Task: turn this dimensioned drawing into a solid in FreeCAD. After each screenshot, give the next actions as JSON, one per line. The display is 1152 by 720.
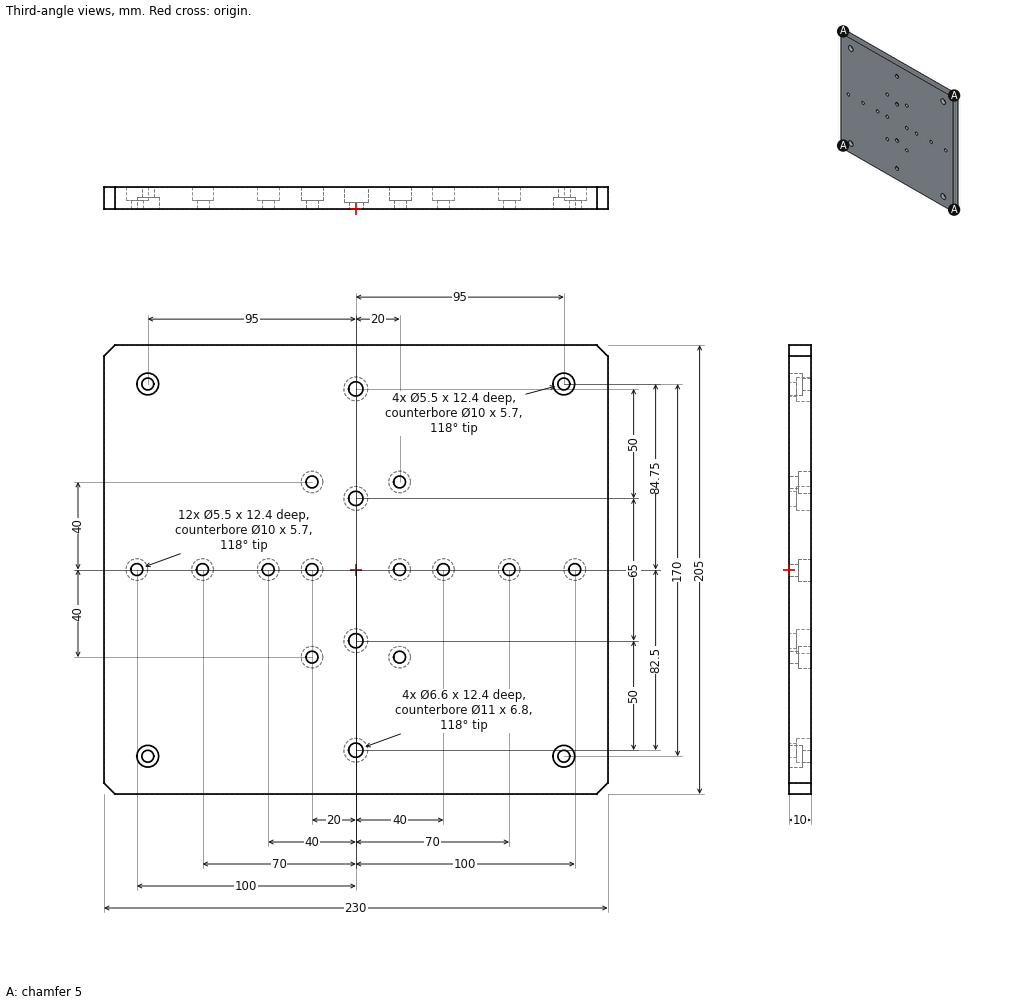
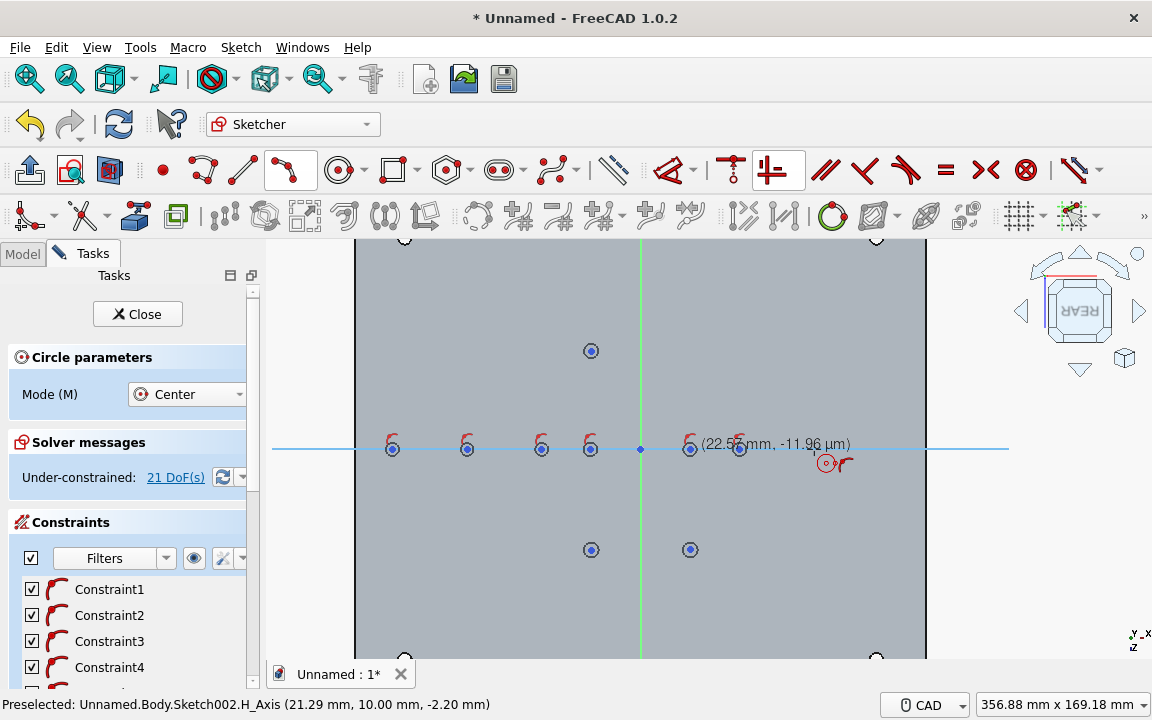
{"action": "left_click", "coordinate": [814, 449]}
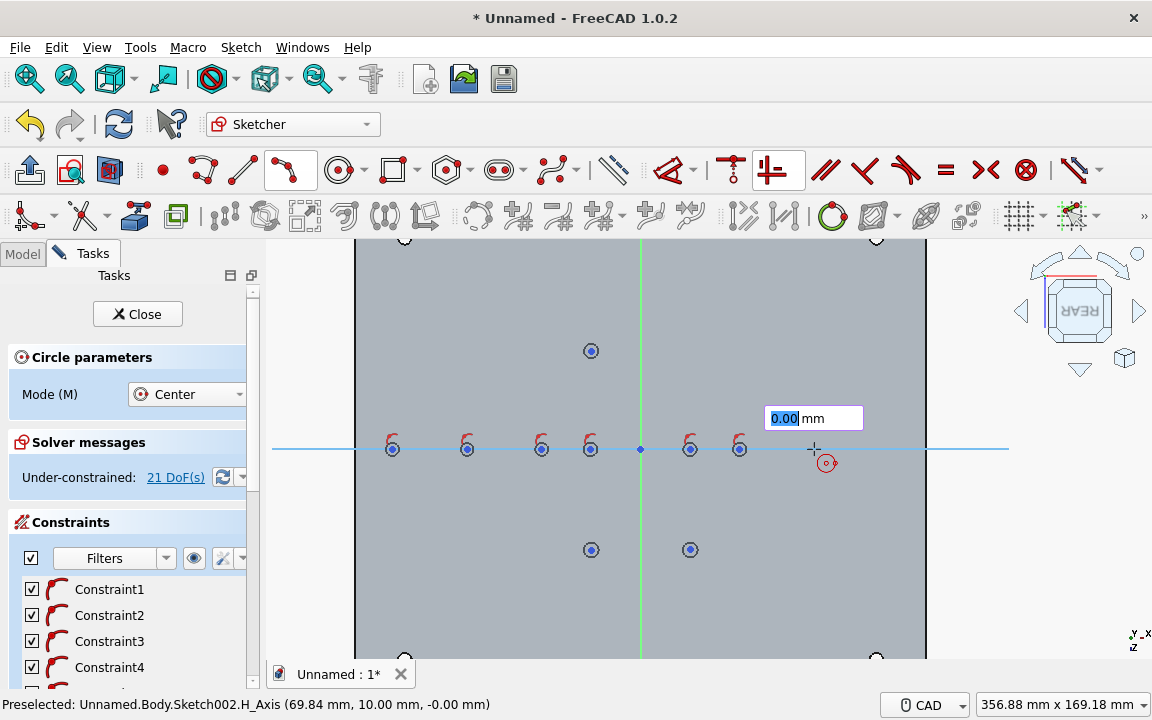
{"action": "scroll", "coordinate": [817, 443], "scroll_direction": "up", "scroll_amount": 5}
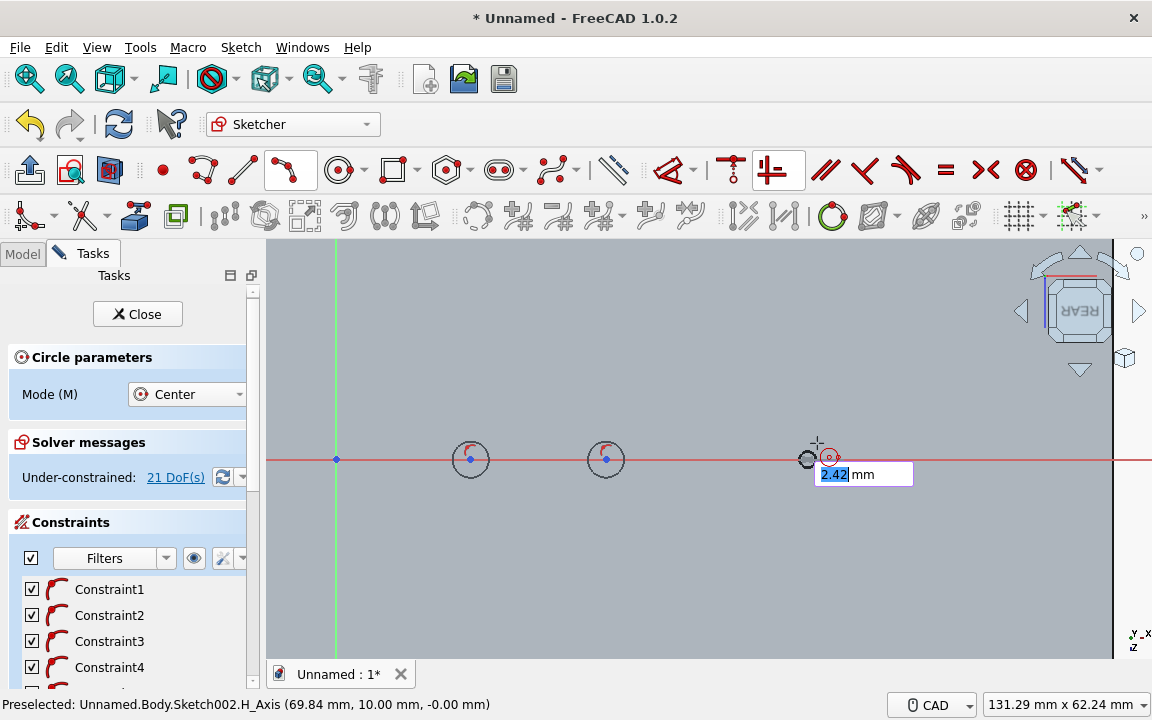
{"action": "left_click", "coordinate": [815, 442]}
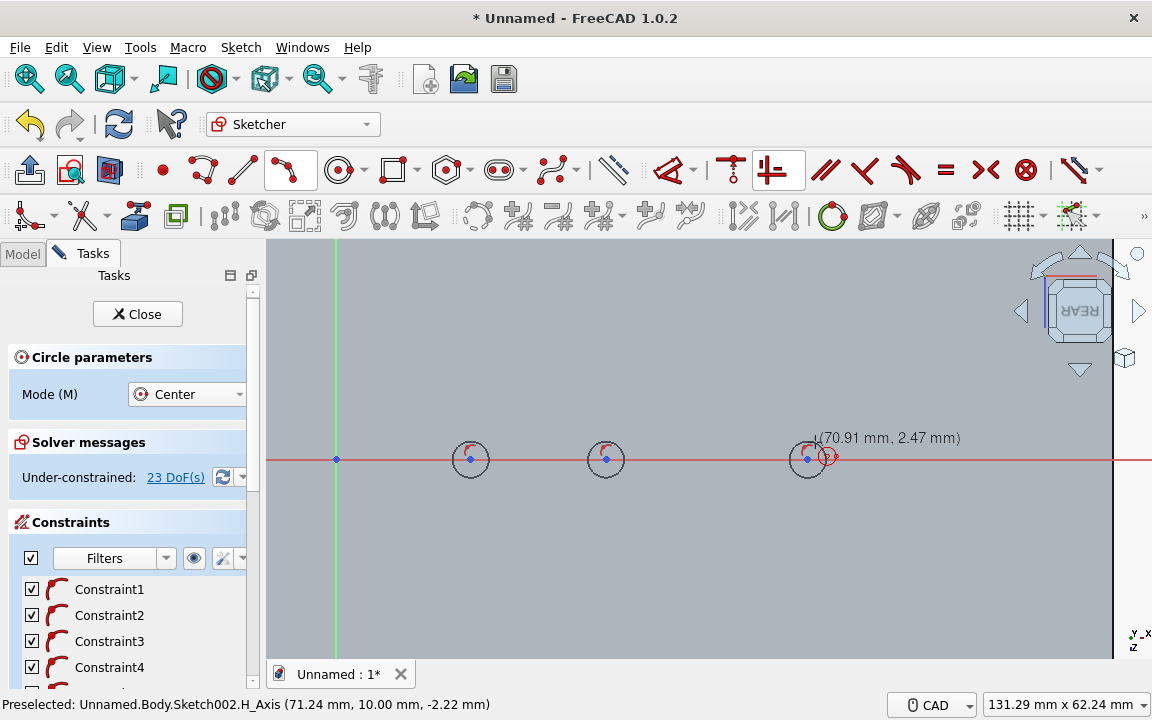
{"action": "scroll", "coordinate": [817, 443], "scroll_direction": "down", "scroll_amount": 5}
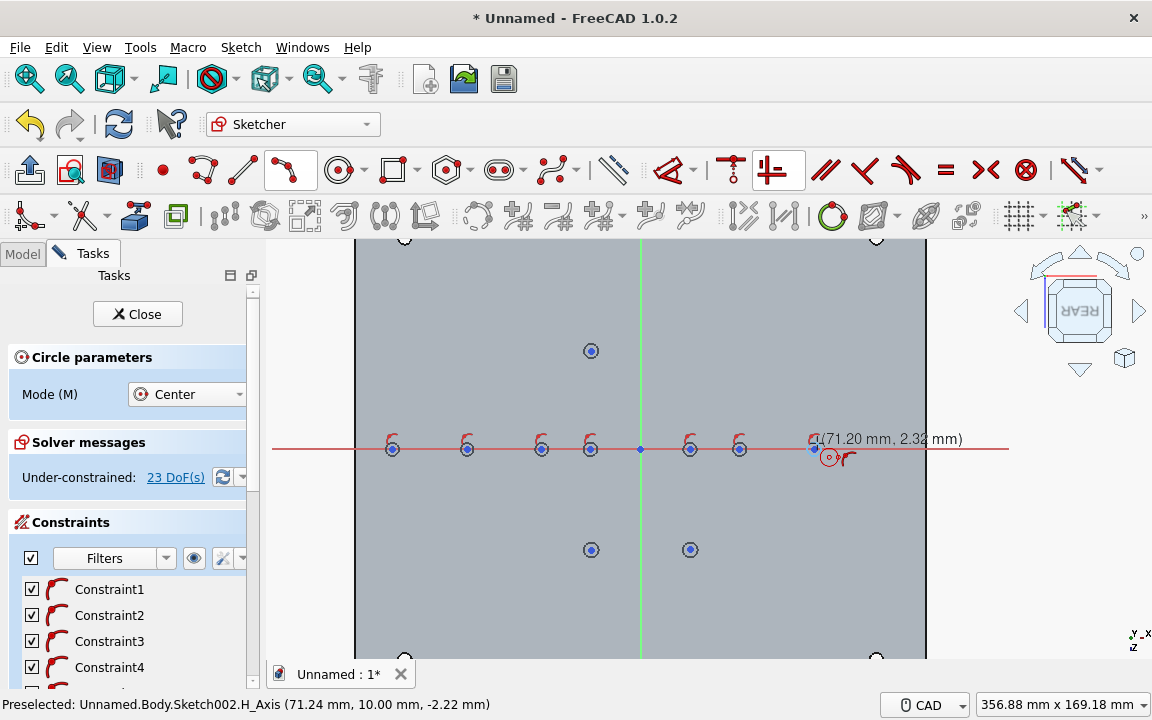
{"action": "scroll", "coordinate": [889, 449], "scroll_direction": "up", "scroll_amount": 7}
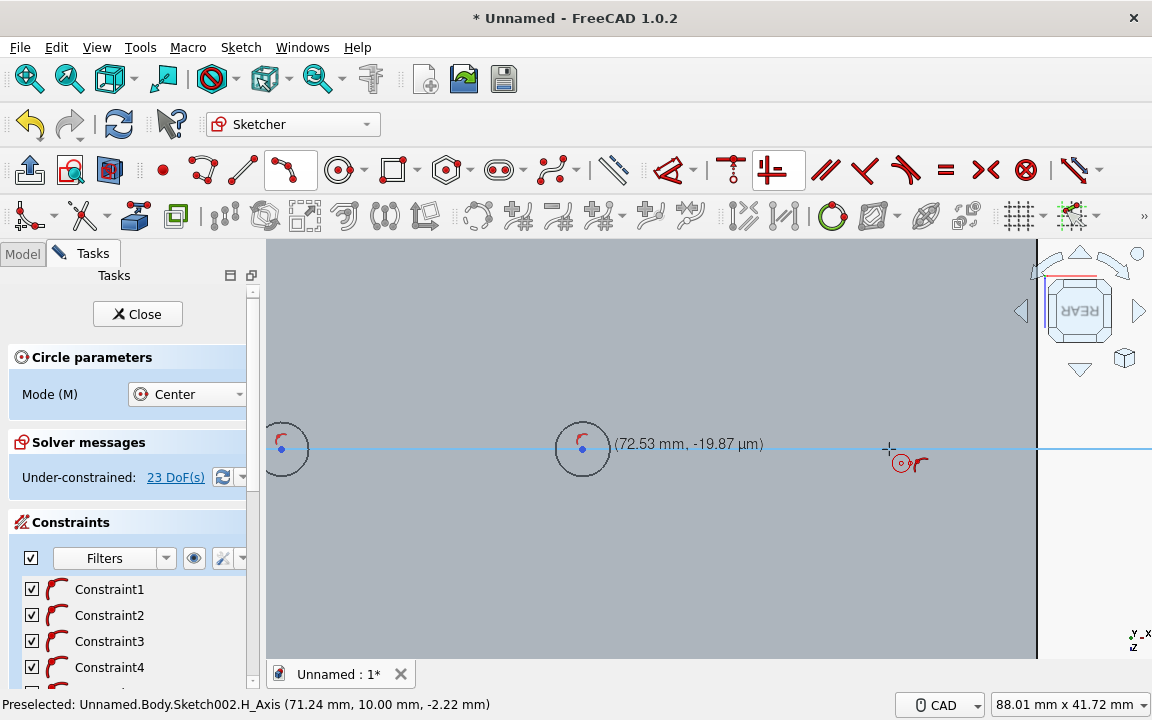
{"action": "scroll", "coordinate": [890, 449], "scroll_direction": "down", "scroll_amount": 7}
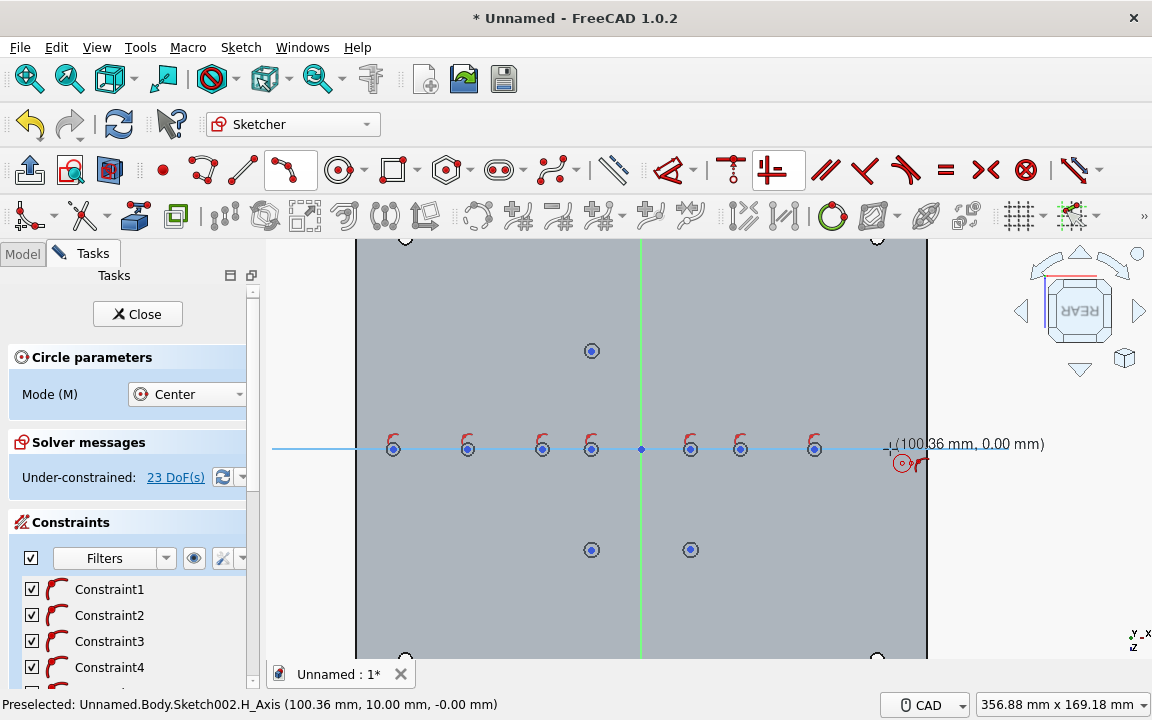
{"action": "left_click", "coordinate": [890, 449]}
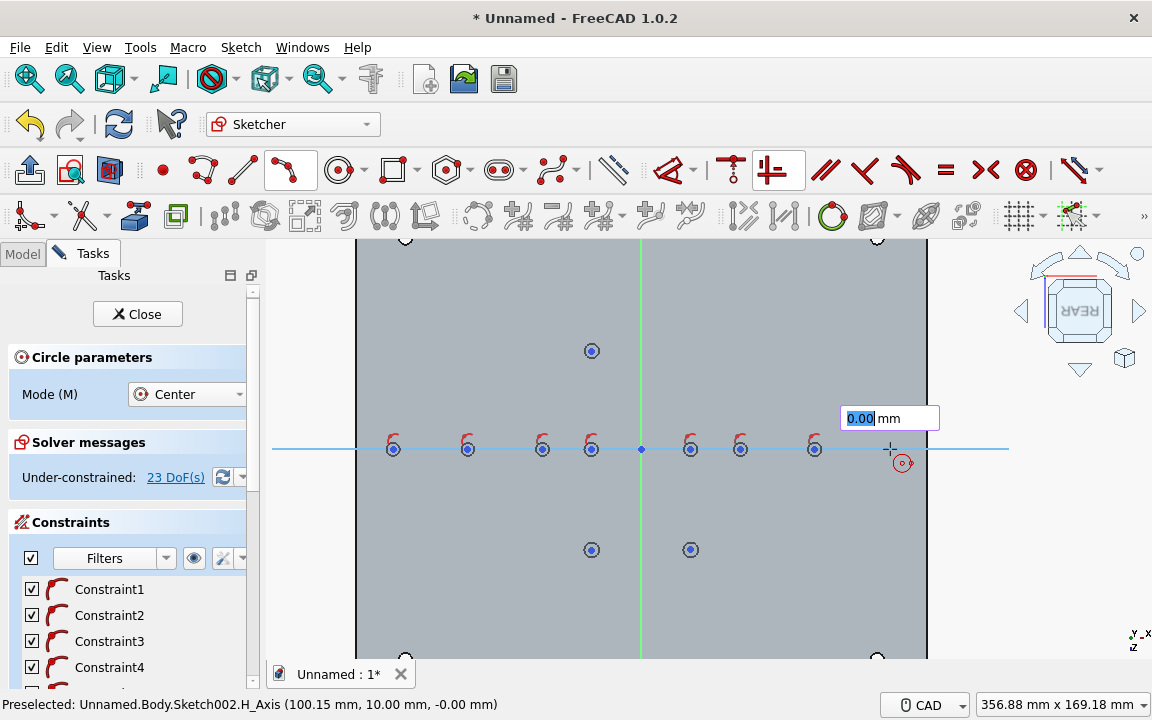
{"action": "scroll", "coordinate": [892, 443], "scroll_direction": "up", "scroll_amount": 5}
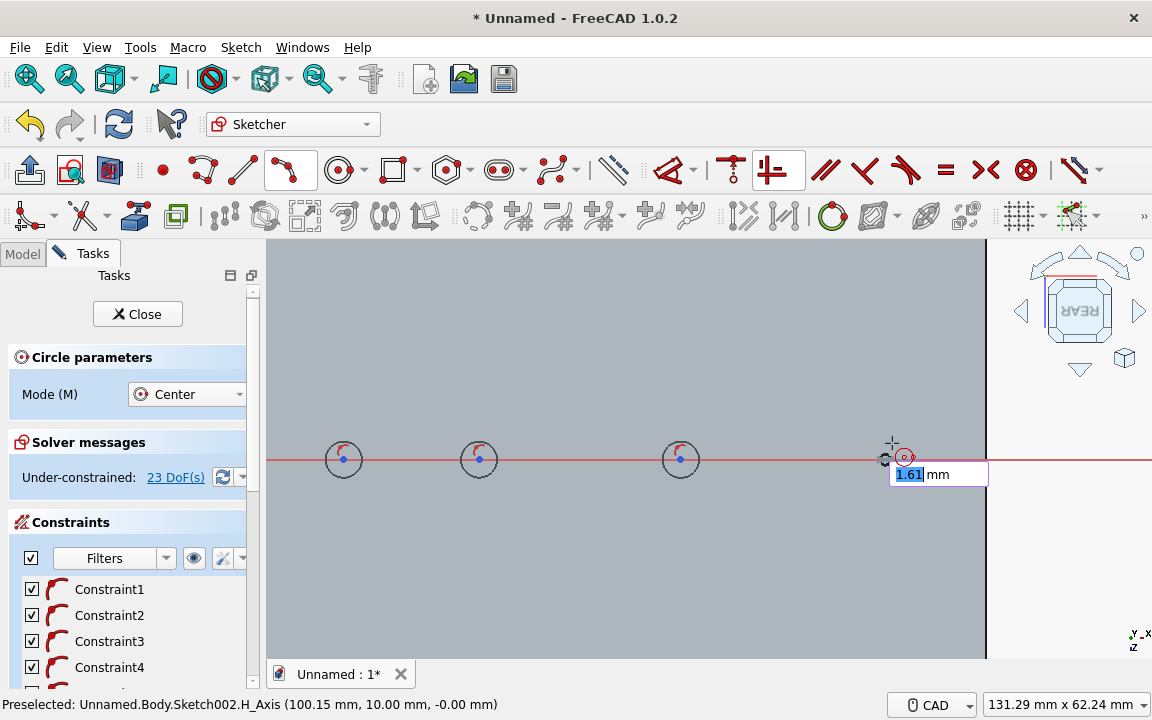
{"action": "left_click", "coordinate": [891, 442]}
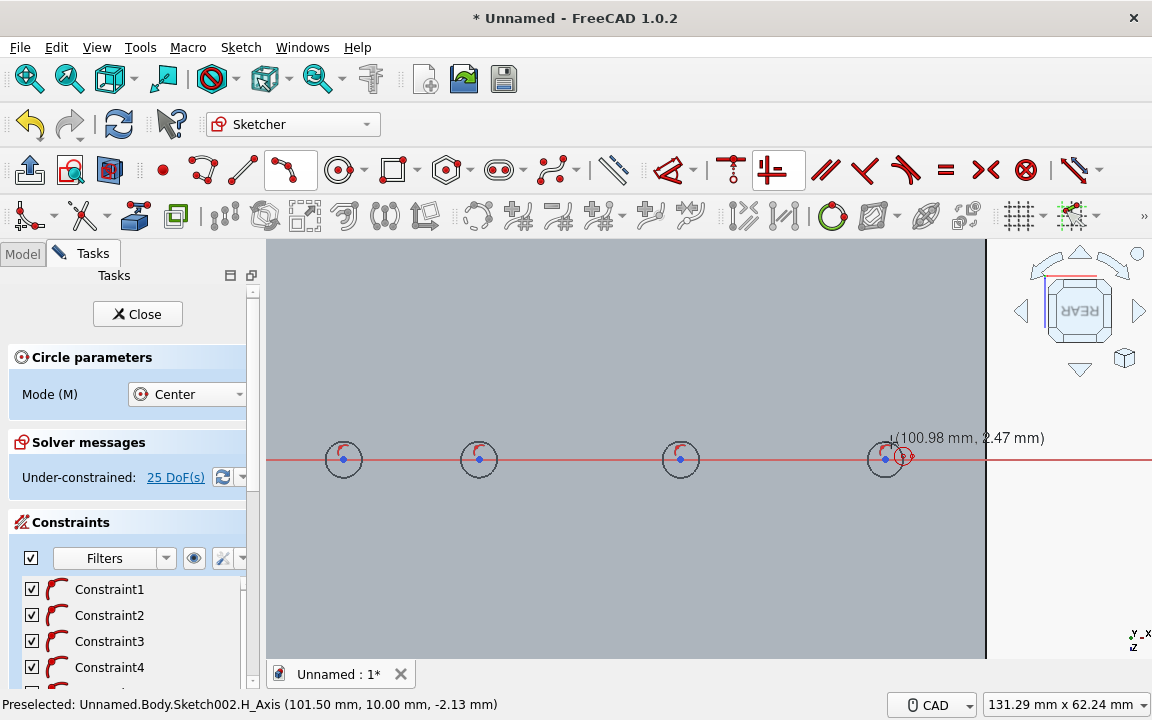
{"action": "scroll", "coordinate": [891, 443], "scroll_direction": "down", "scroll_amount": 5}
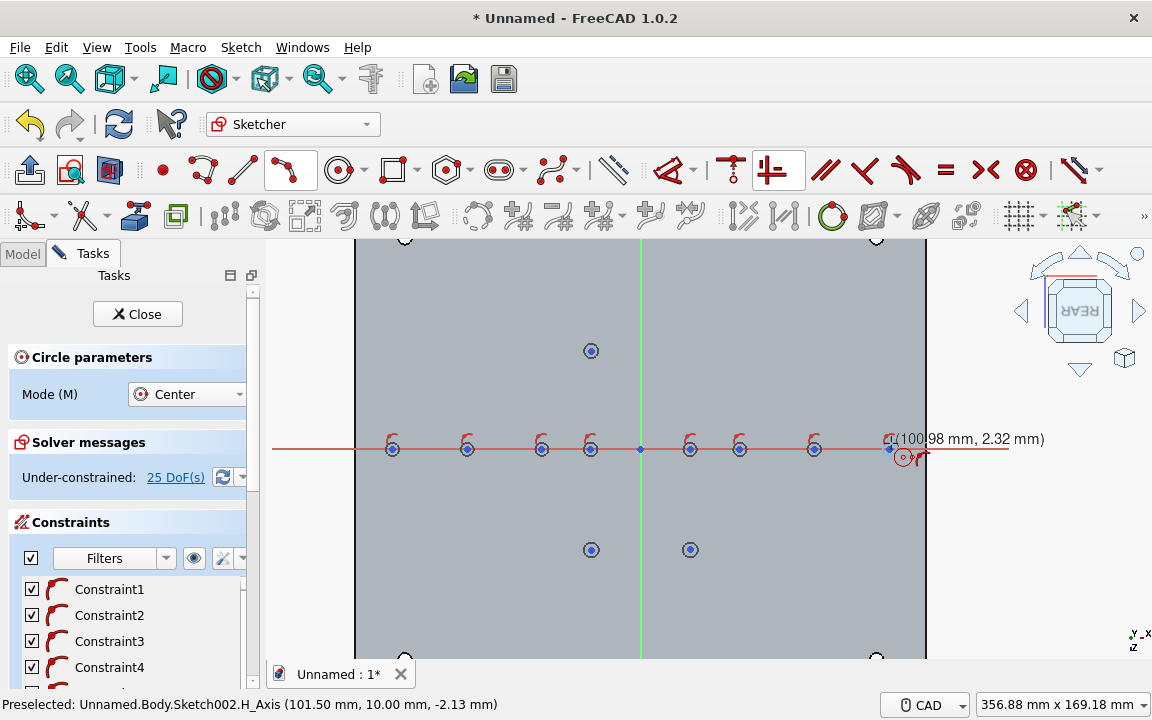
{"action": "scroll", "coordinate": [690, 350], "scroll_direction": "up", "scroll_amount": 7}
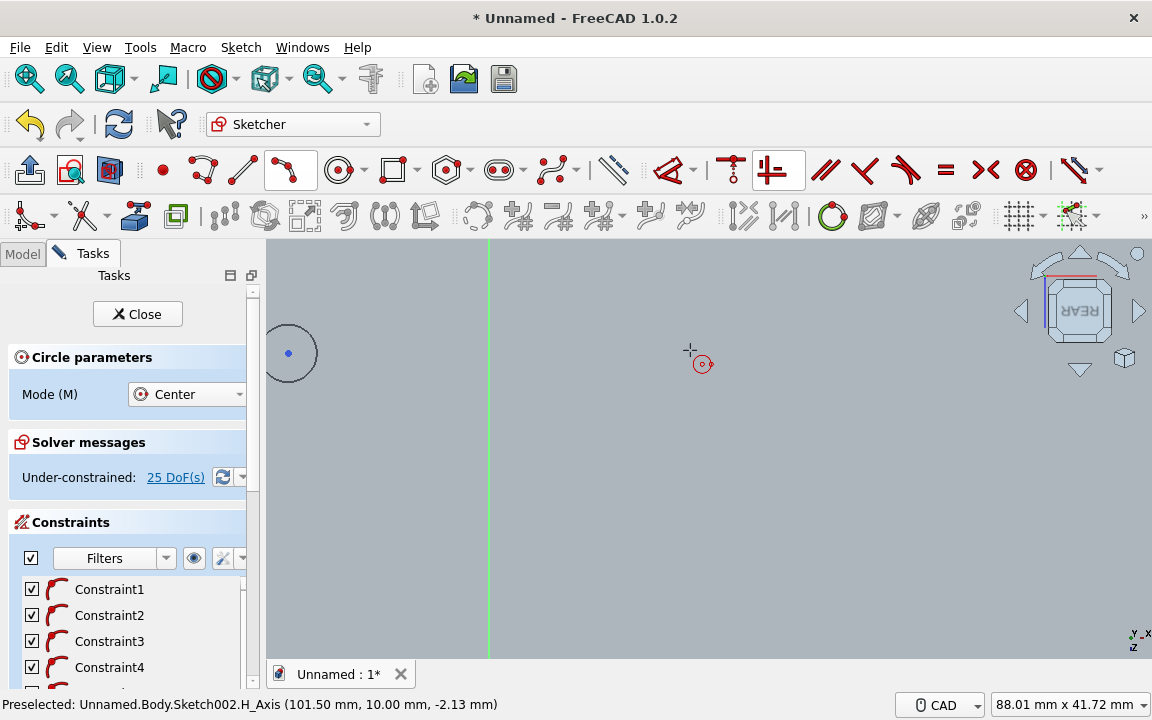
{"action": "scroll", "coordinate": [690, 350], "scroll_direction": "down", "scroll_amount": 7}